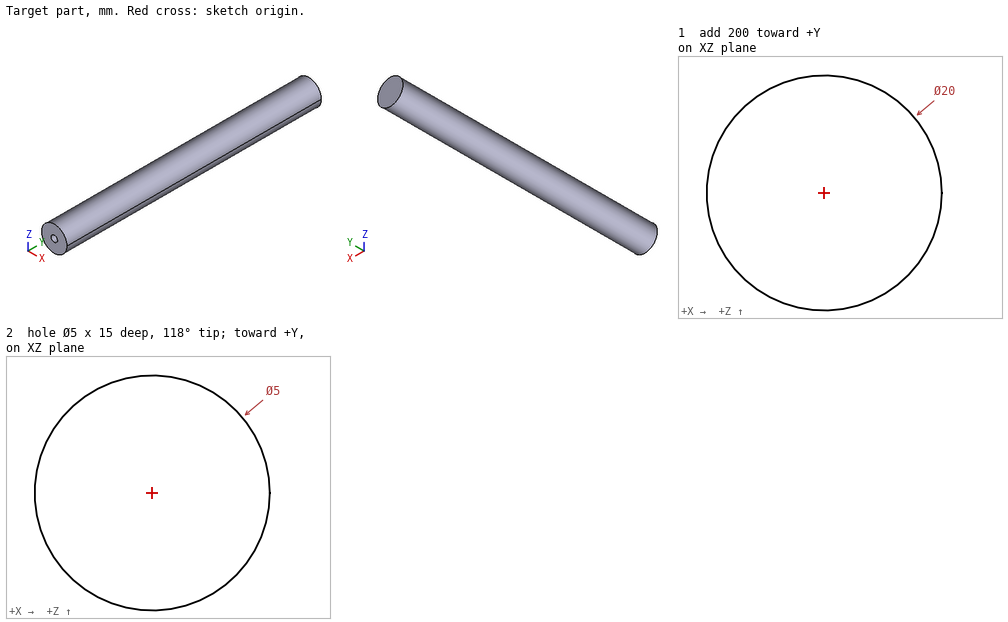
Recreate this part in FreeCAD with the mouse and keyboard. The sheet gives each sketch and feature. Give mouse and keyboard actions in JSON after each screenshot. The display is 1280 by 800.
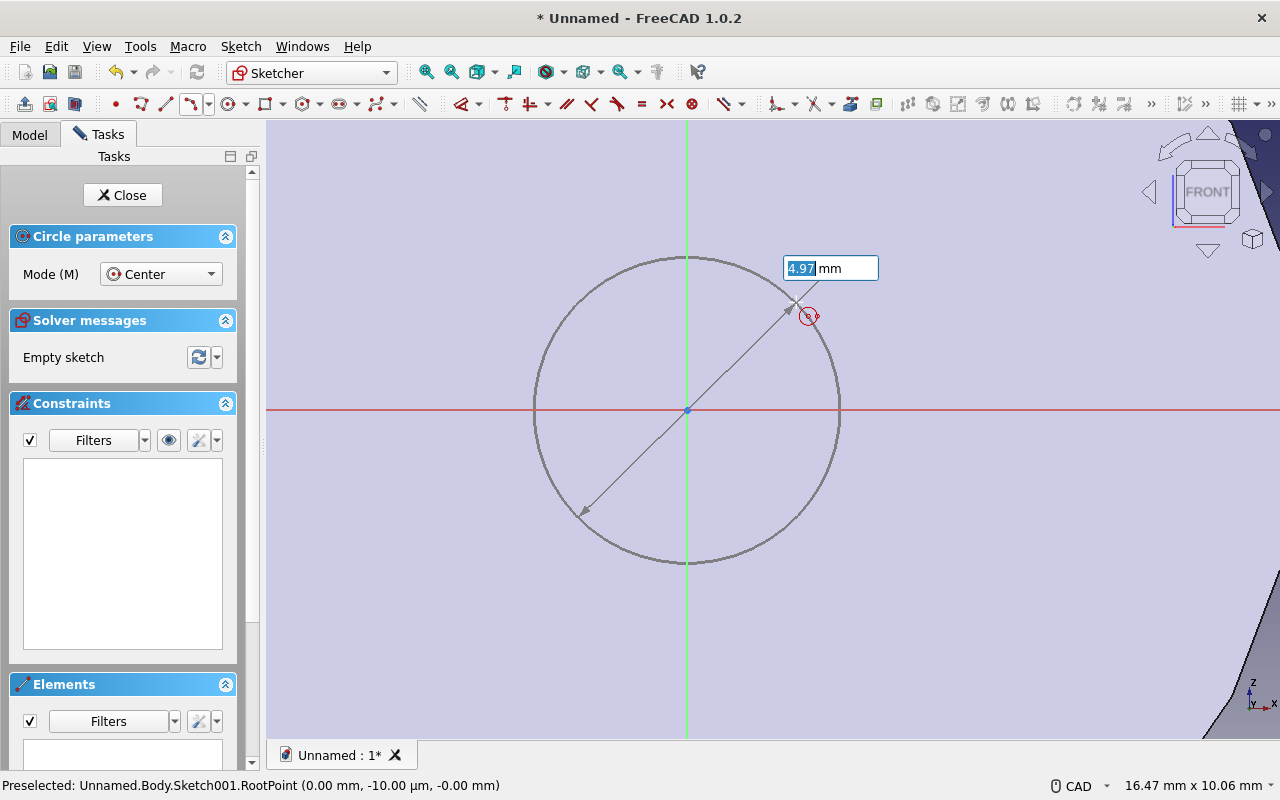
{"action": "type", "text": "5"}
{"action": "key", "text": "Return"}
{"action": "key", "text": "Escape"}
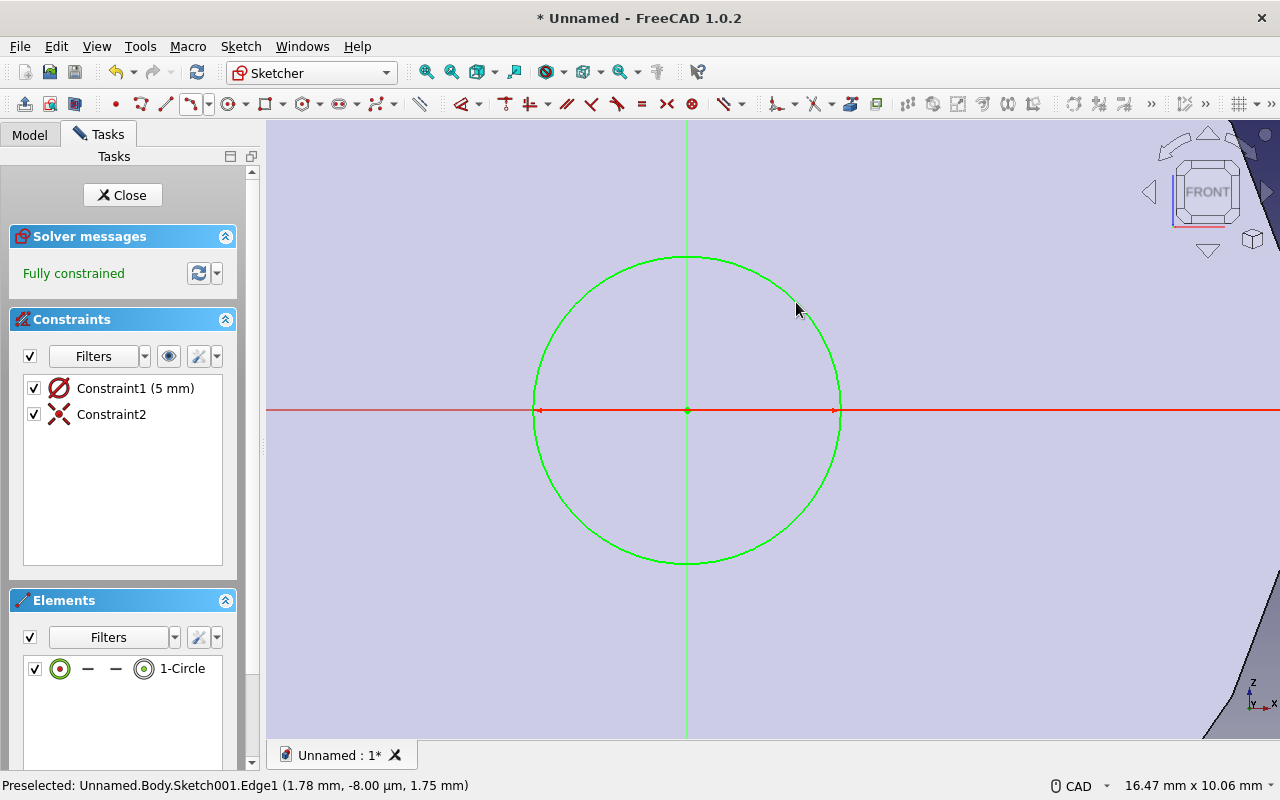
{"action": "left_click", "coordinate": [123, 195]}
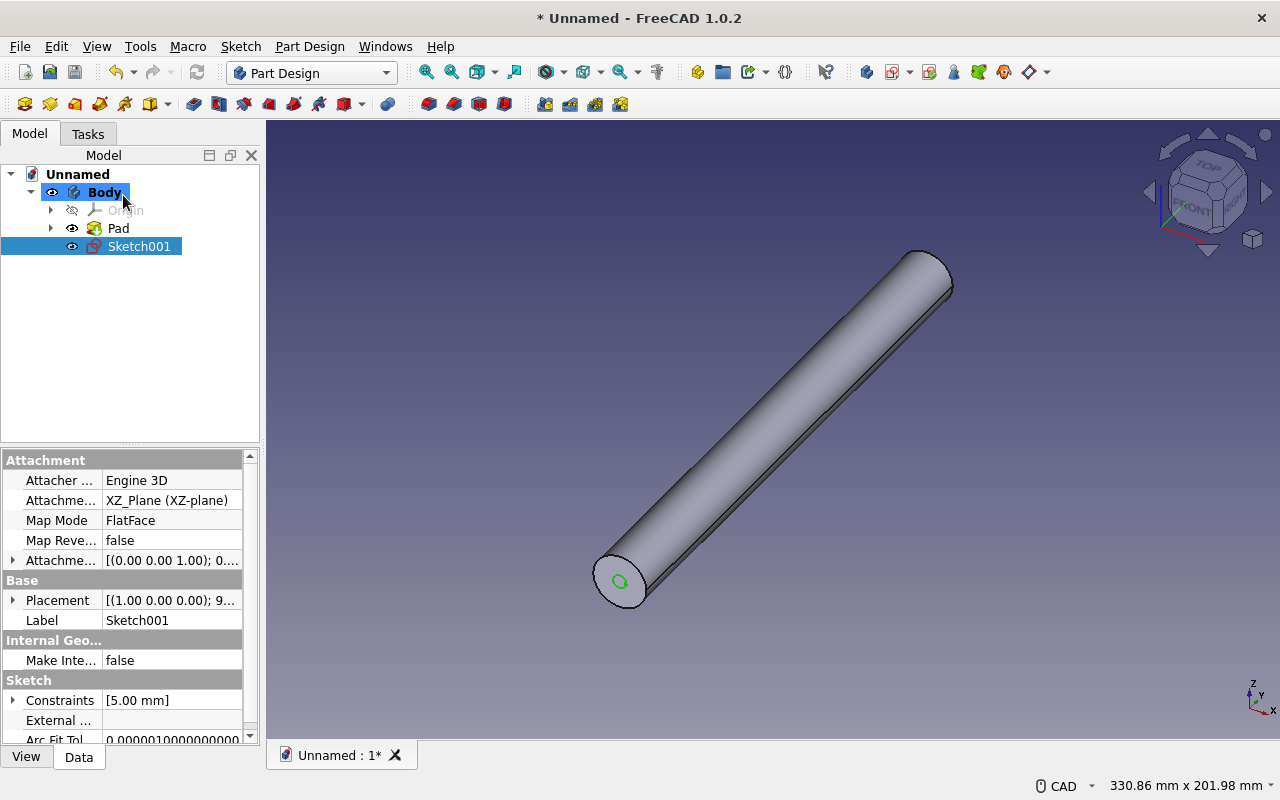
{"action": "left_click", "coordinate": [219, 104]}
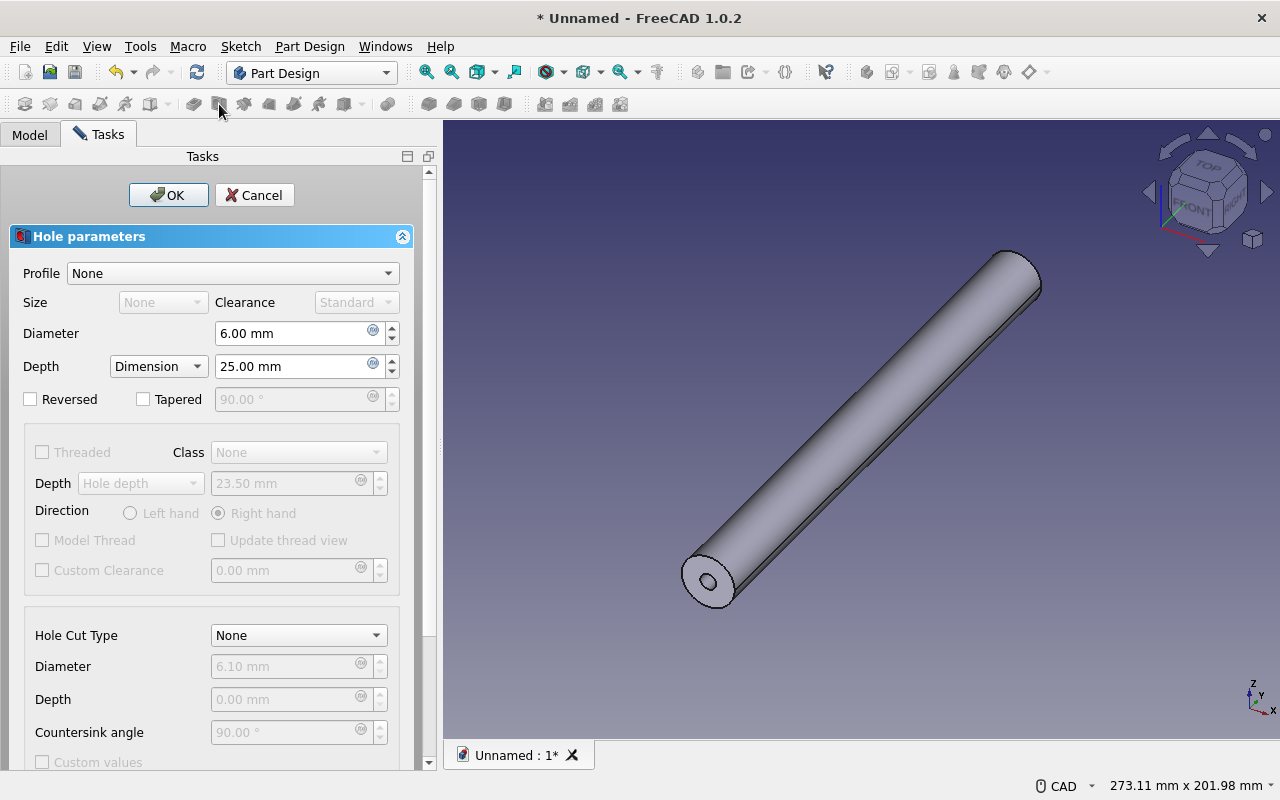
{"action": "triple_click", "coordinate": [300, 334]}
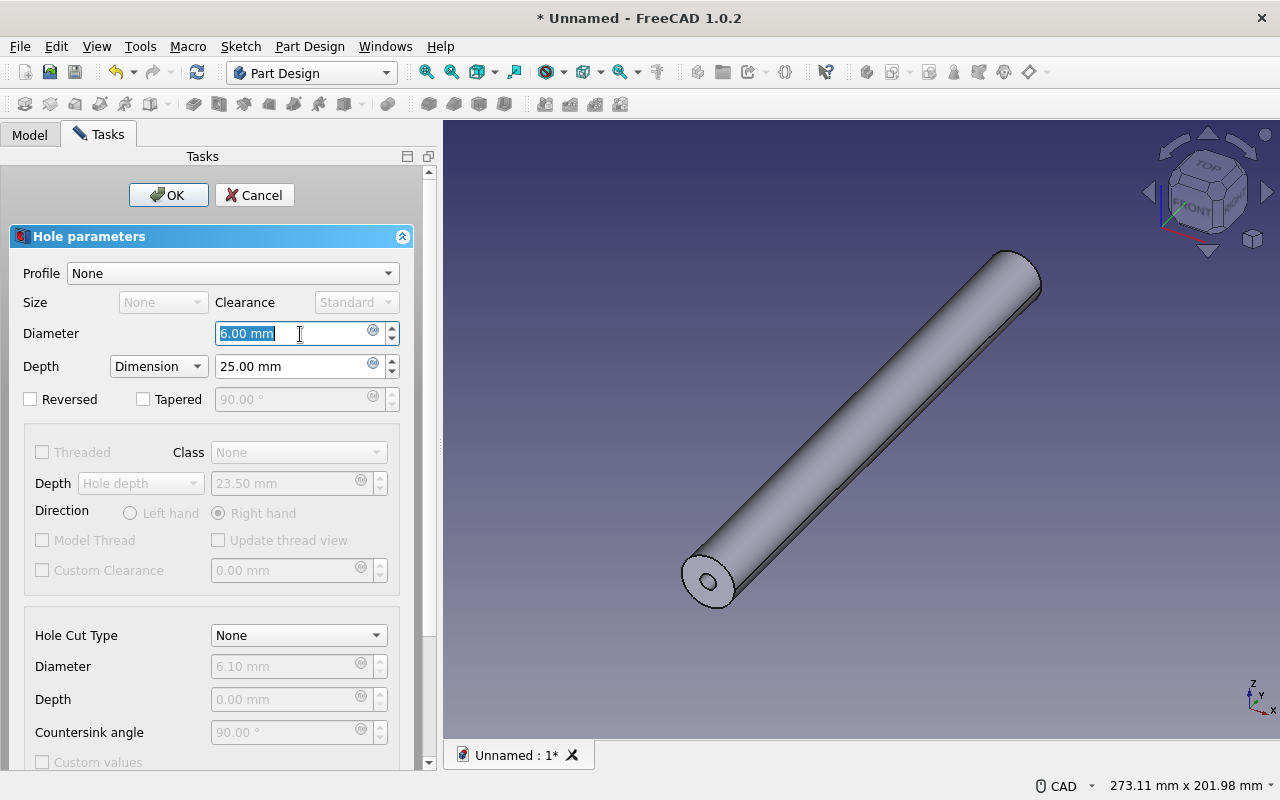
{"action": "type", "text": "5"}
{"action": "key", "text": "Tab"}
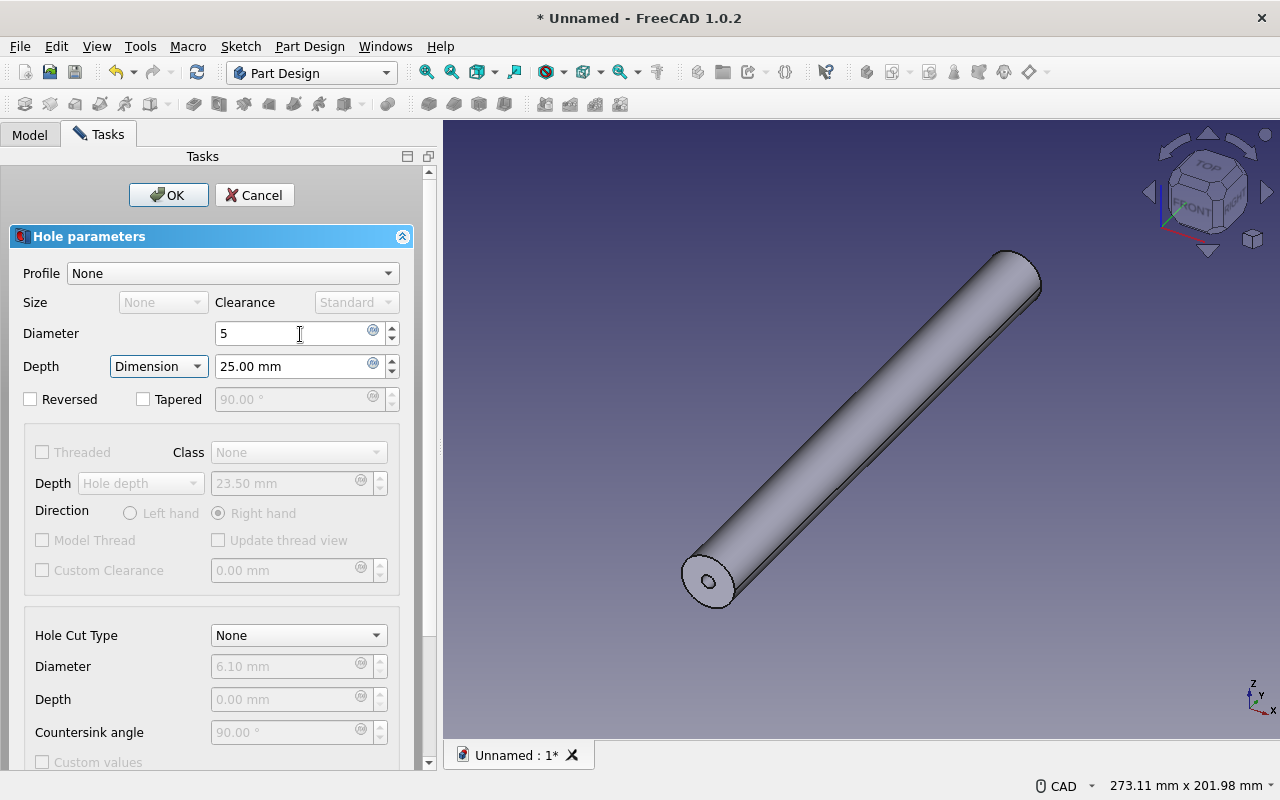
{"action": "triple_click", "coordinate": [300, 366]}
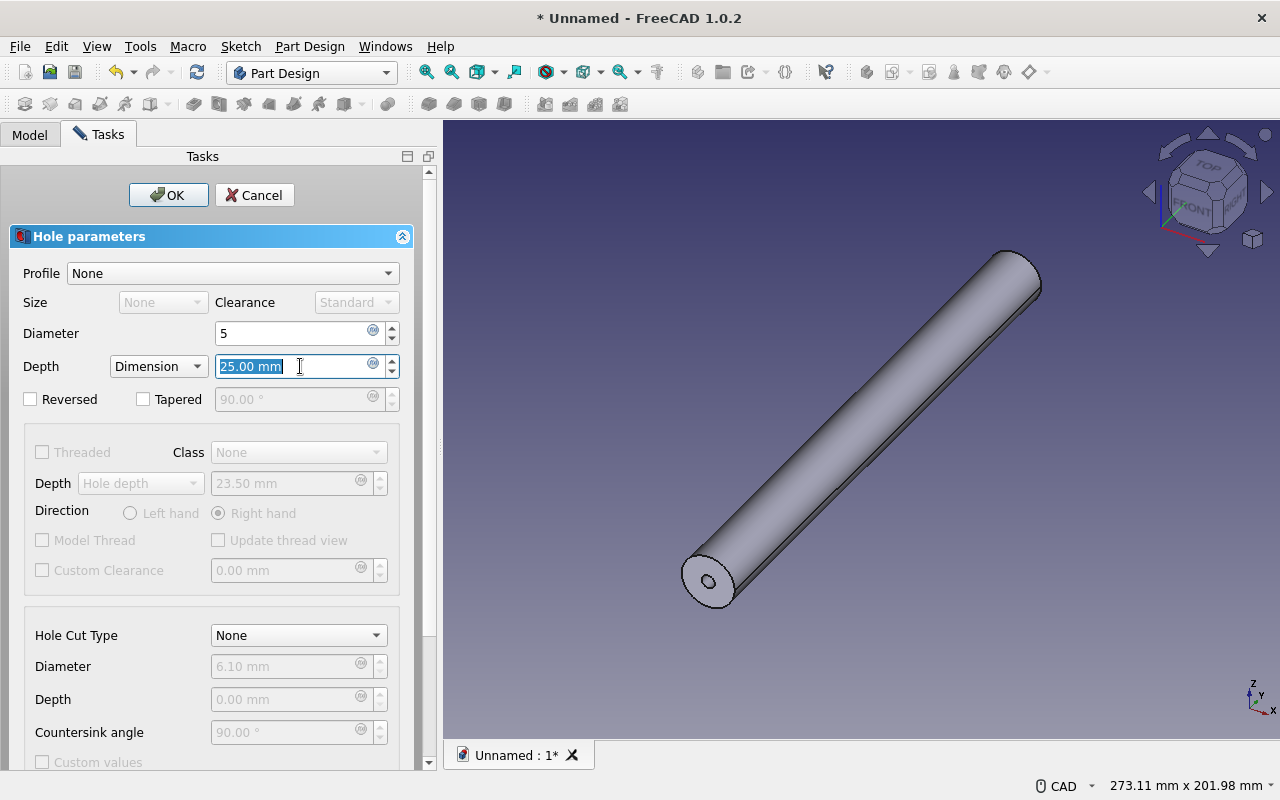
{"action": "type", "text": "15"}
{"action": "key", "text": "Tab"}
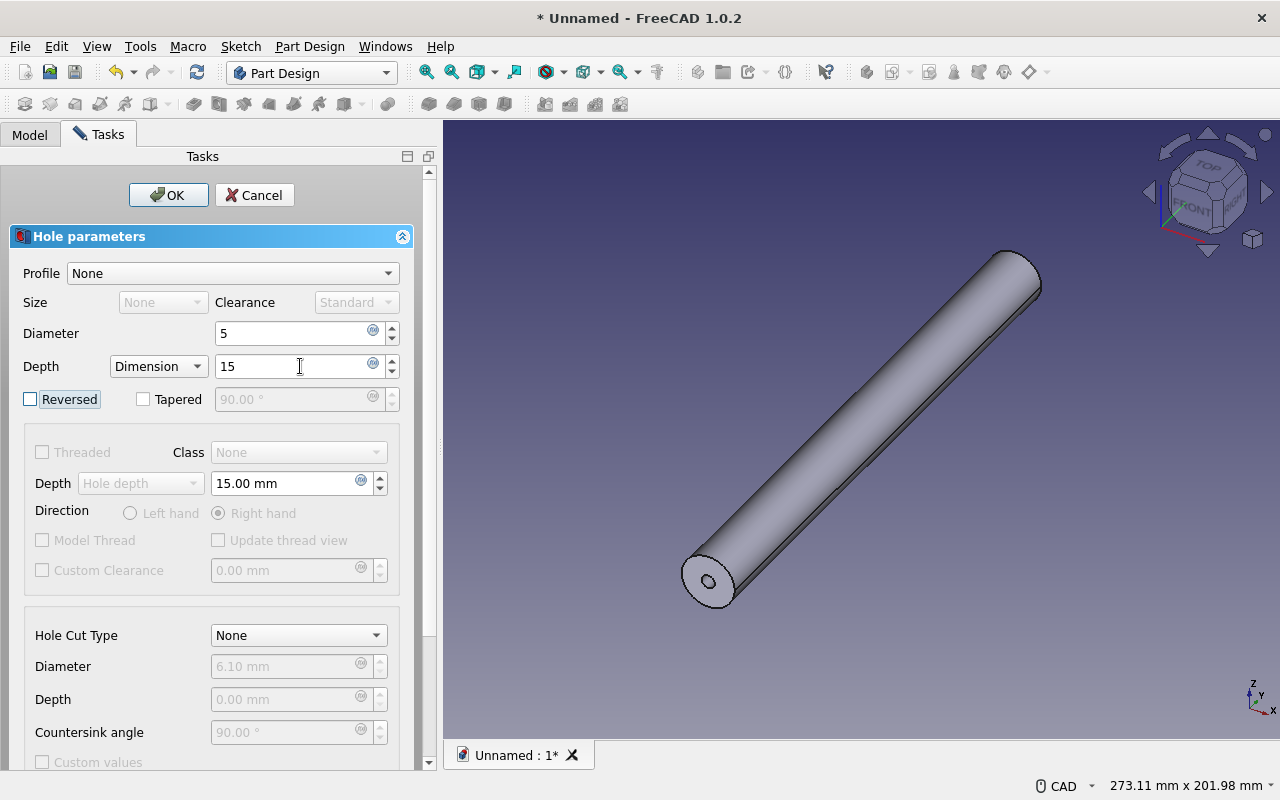
{"action": "left_click", "coordinate": [169, 195]}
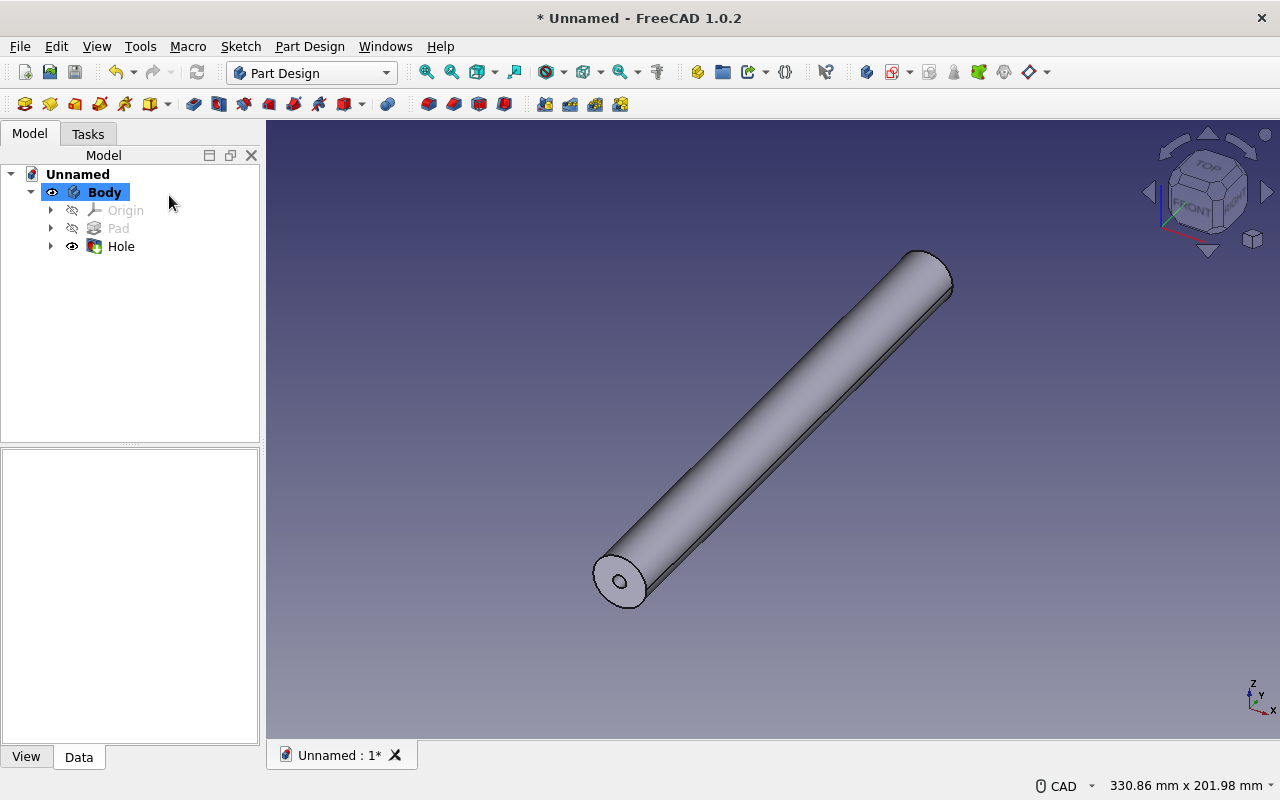
{"action": "key", "text": "0"}